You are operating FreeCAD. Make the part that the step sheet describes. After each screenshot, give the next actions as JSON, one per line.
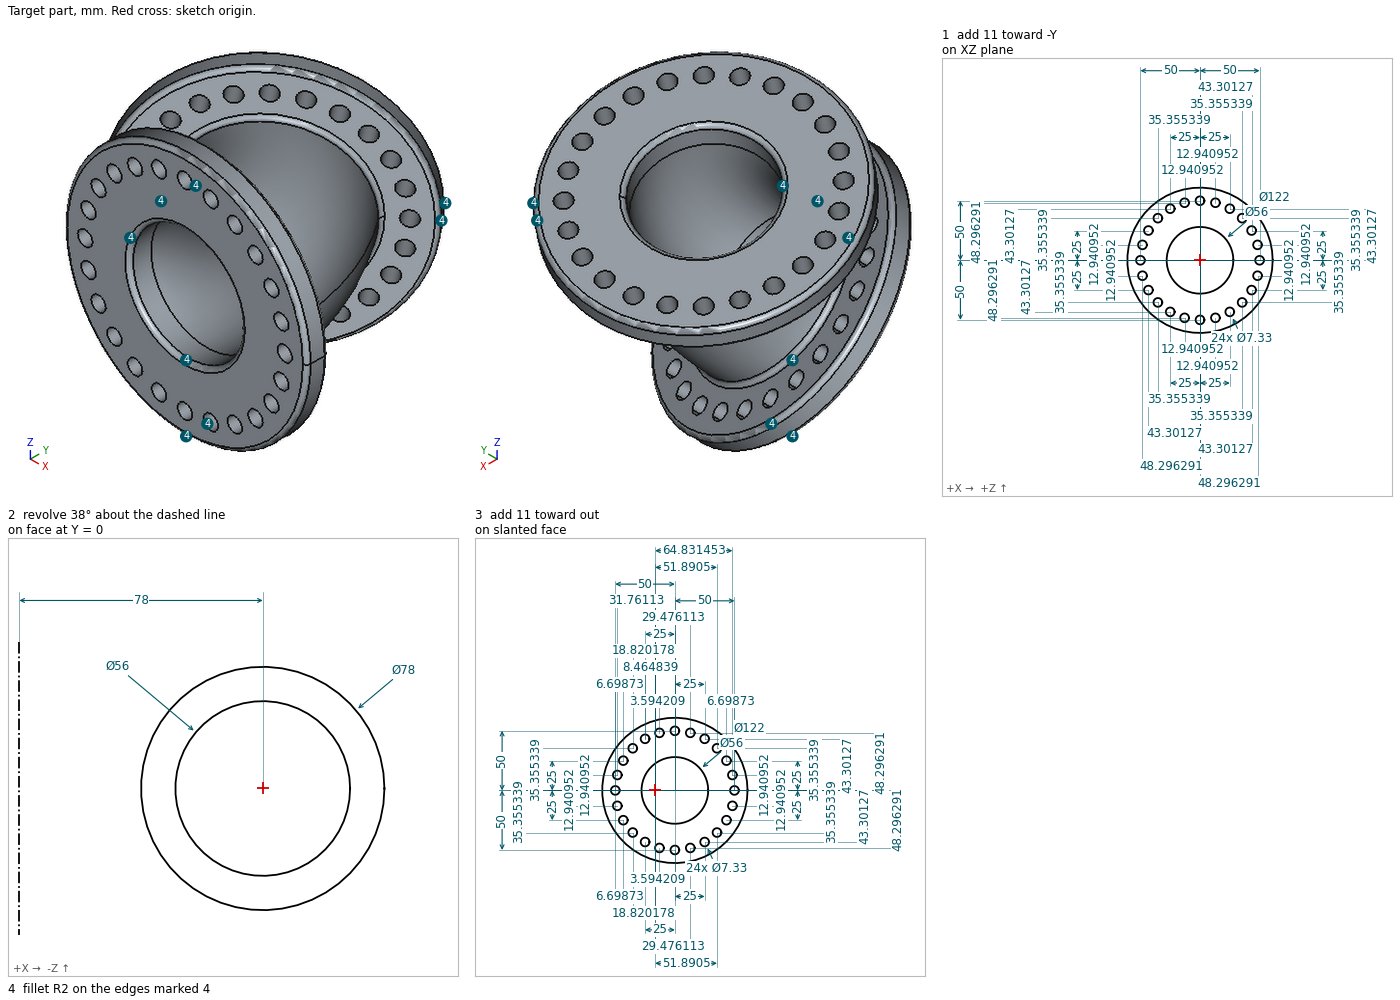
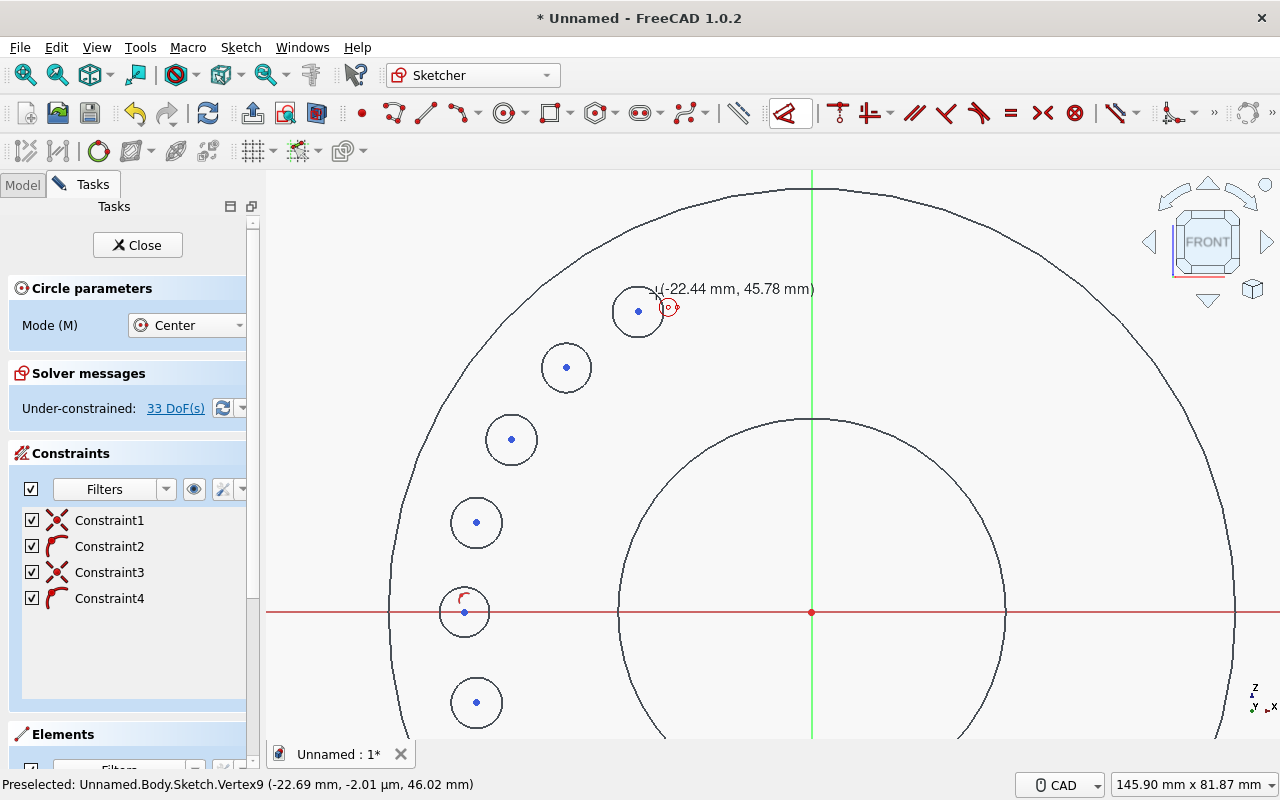
{"action": "left_click", "coordinate": [722, 277]}
{"action": "left_click", "coordinate": [740, 259]}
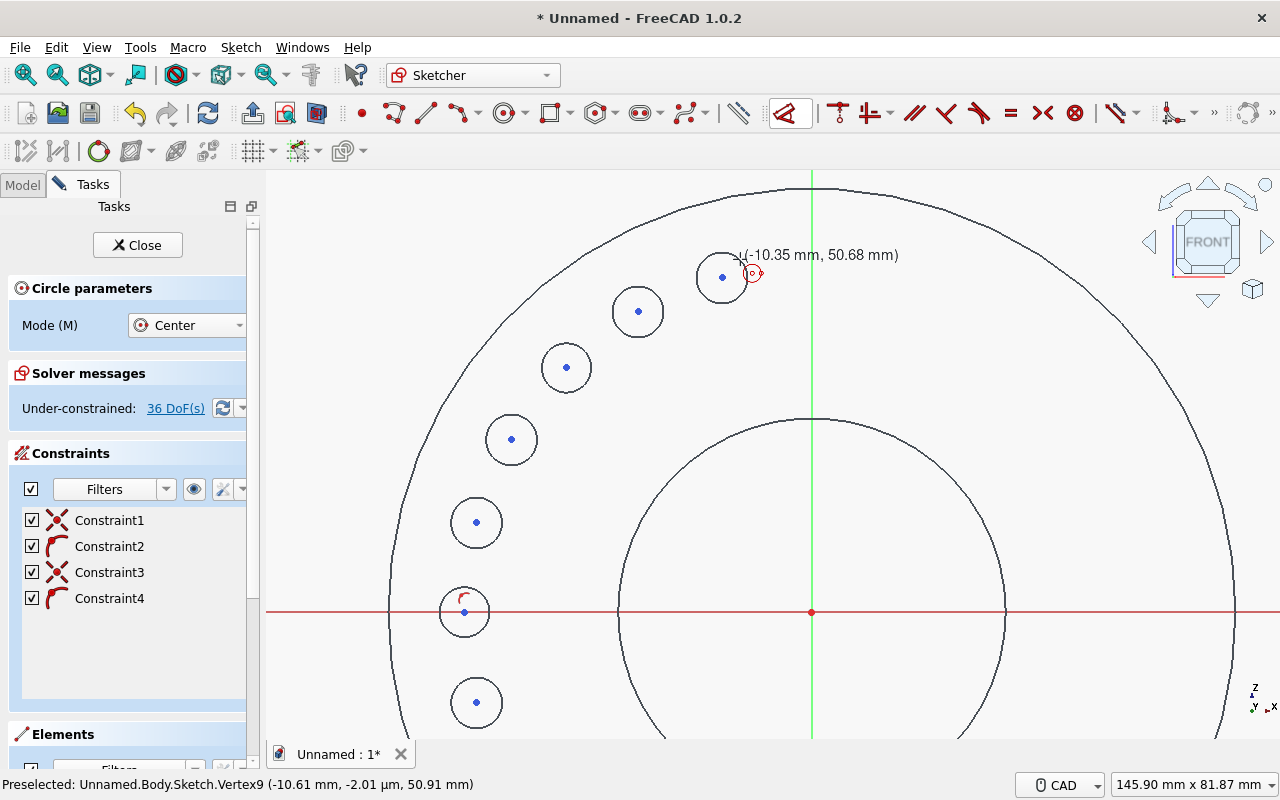
{"action": "scroll", "coordinate": [617, 326], "scroll_direction": "down", "scroll_amount": 4}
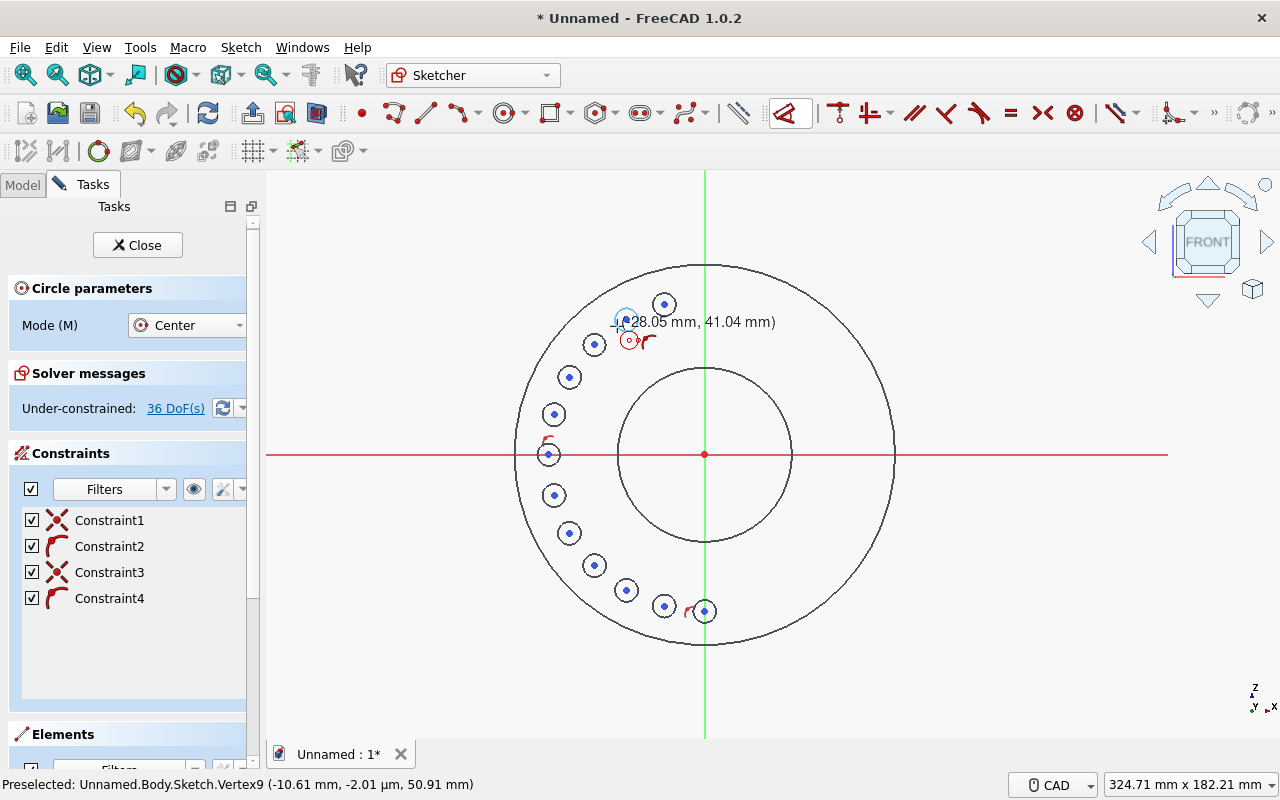
{"action": "scroll", "coordinate": [745, 606], "scroll_direction": "up", "scroll_amount": 4}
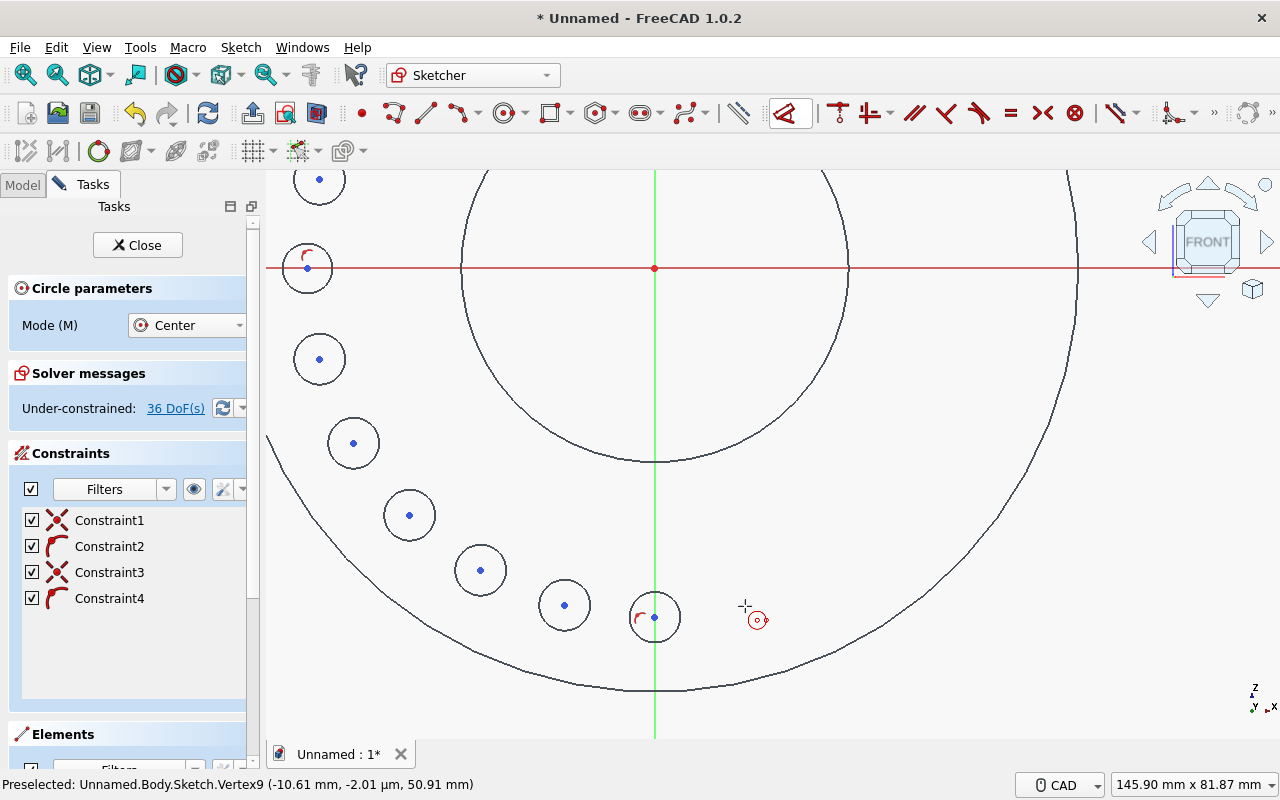
{"action": "left_click", "coordinate": [745, 604]}
{"action": "left_click", "coordinate": [763, 586]}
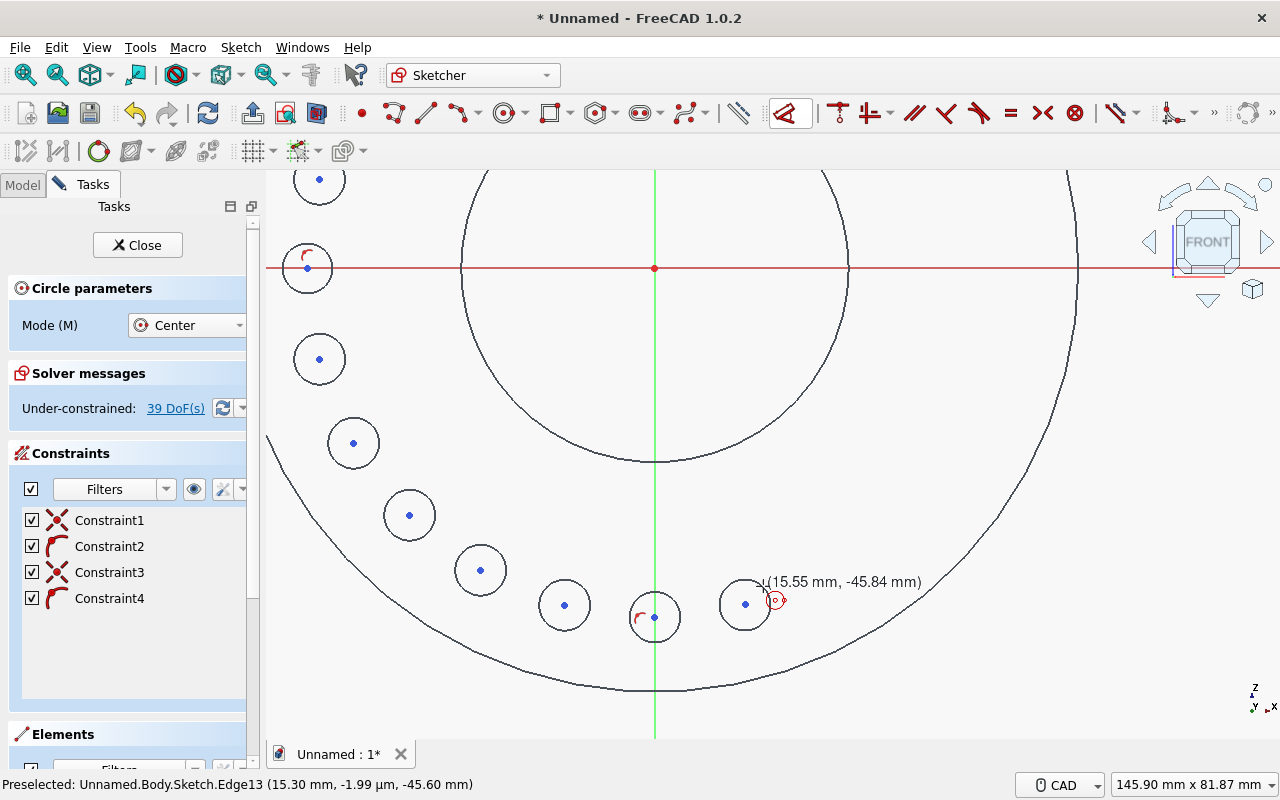
{"action": "left_click", "coordinate": [829, 569]}
{"action": "left_click", "coordinate": [847, 551]}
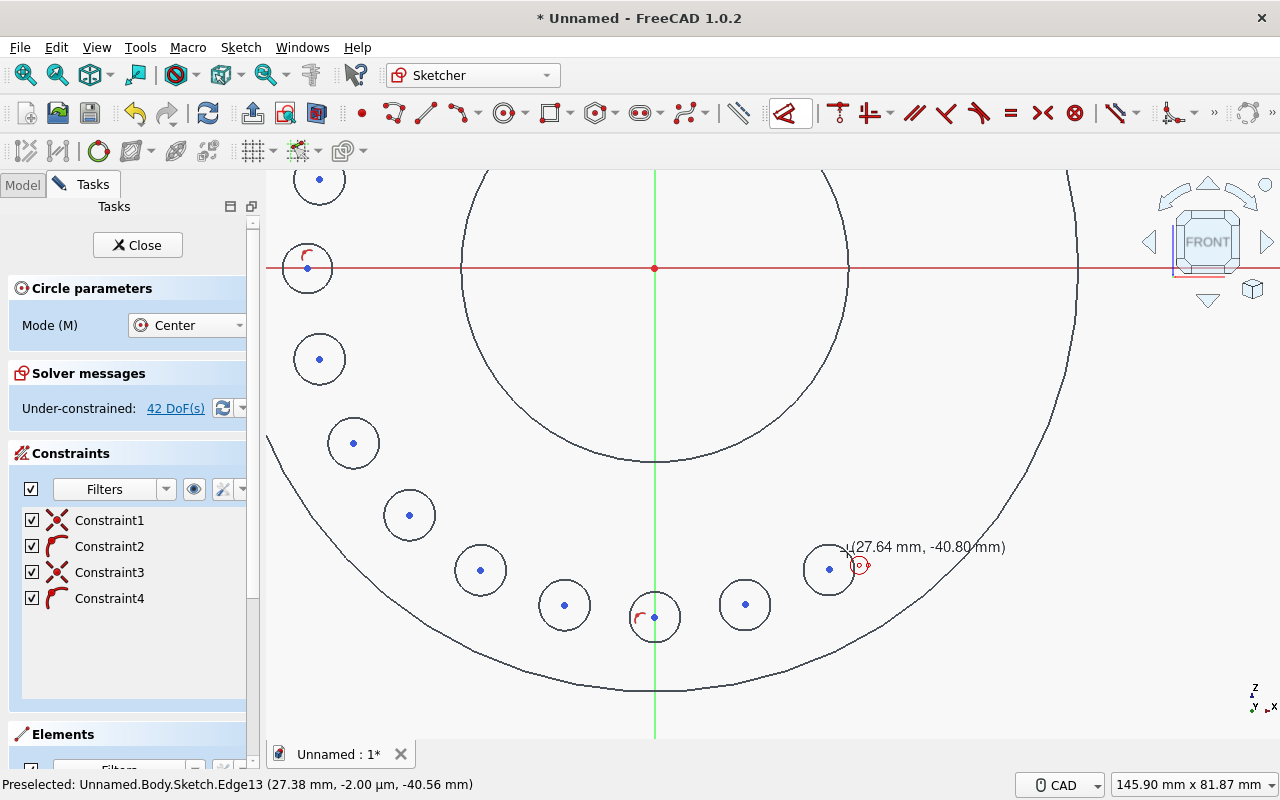
{"action": "left_click", "coordinate": [901, 514]}
{"action": "left_click", "coordinate": [919, 496]}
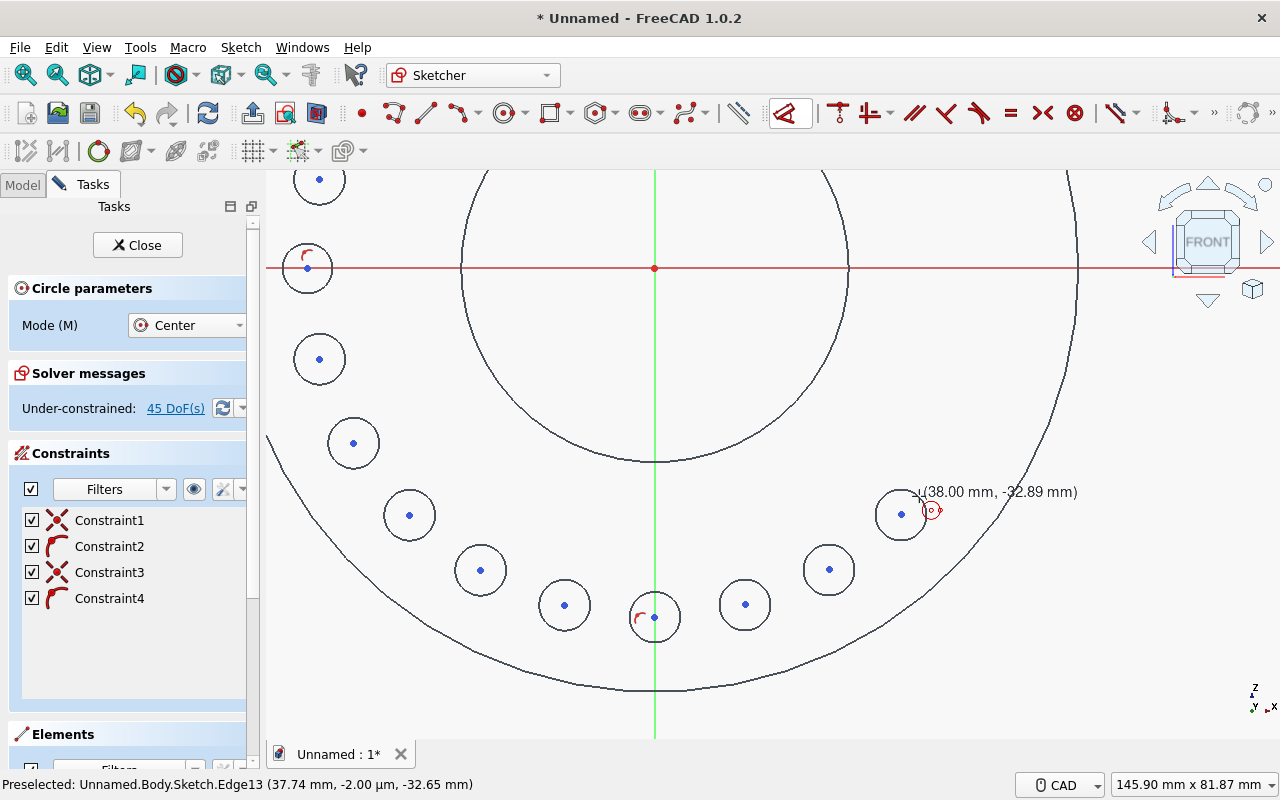
{"action": "left_click", "coordinate": [956, 442]}
{"action": "left_click", "coordinate": [974, 424]}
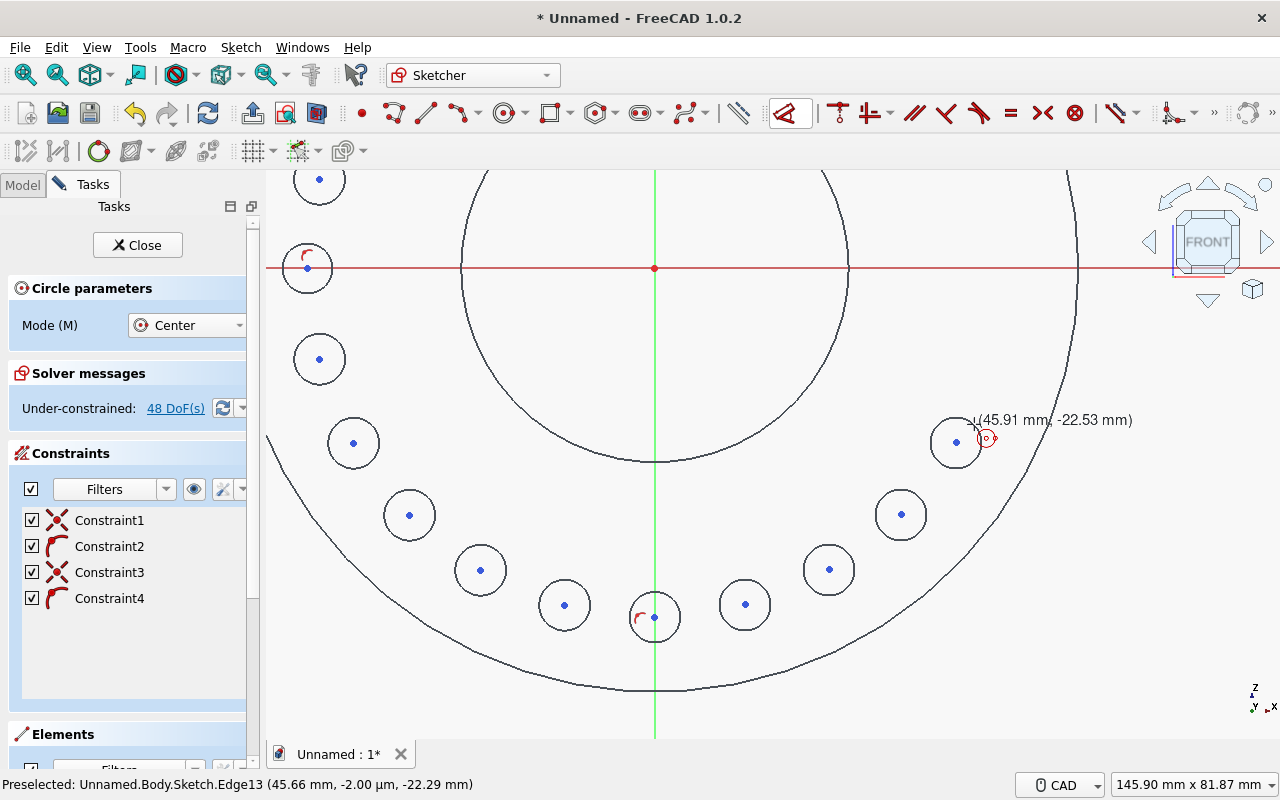
{"action": "left_click", "coordinate": [991, 358]}
{"action": "left_click", "coordinate": [1009, 340]}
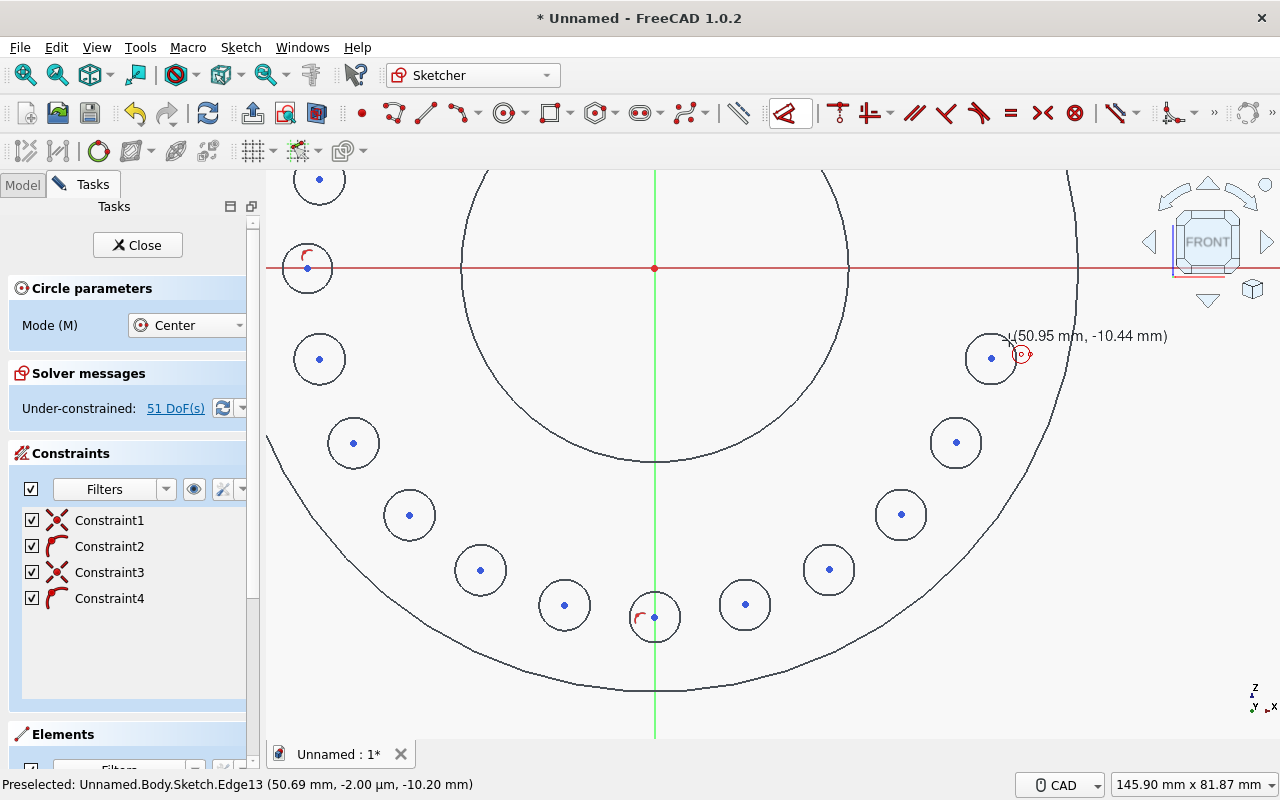
{"action": "left_click", "coordinate": [1002, 268]}
{"action": "left_click", "coordinate": [1020, 250]}